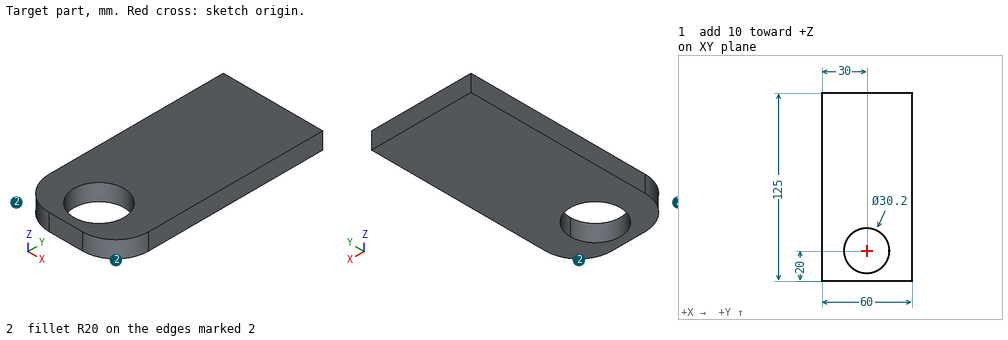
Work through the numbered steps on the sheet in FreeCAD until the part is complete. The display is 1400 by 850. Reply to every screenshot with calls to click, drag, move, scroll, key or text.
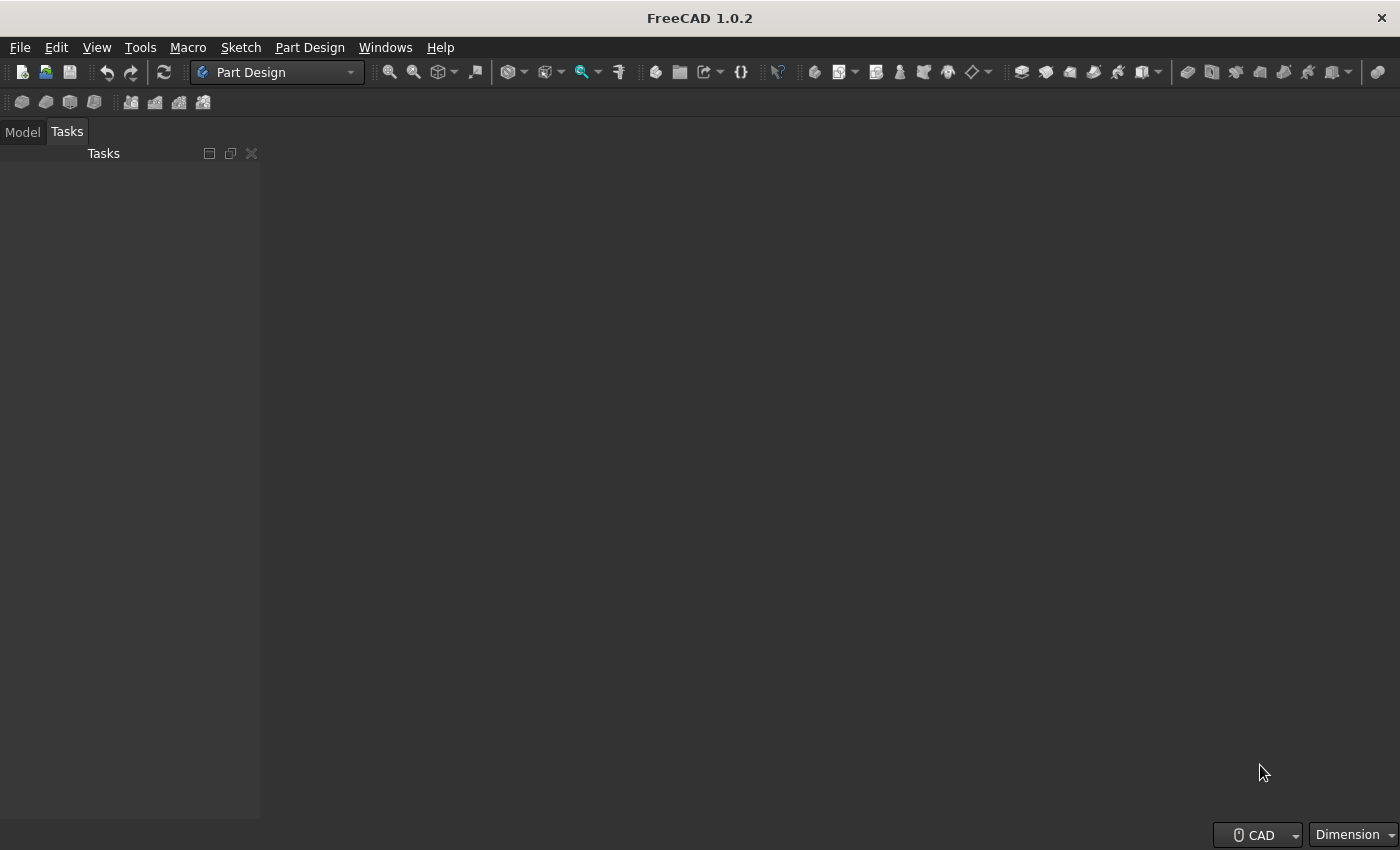
key(ctrl+n)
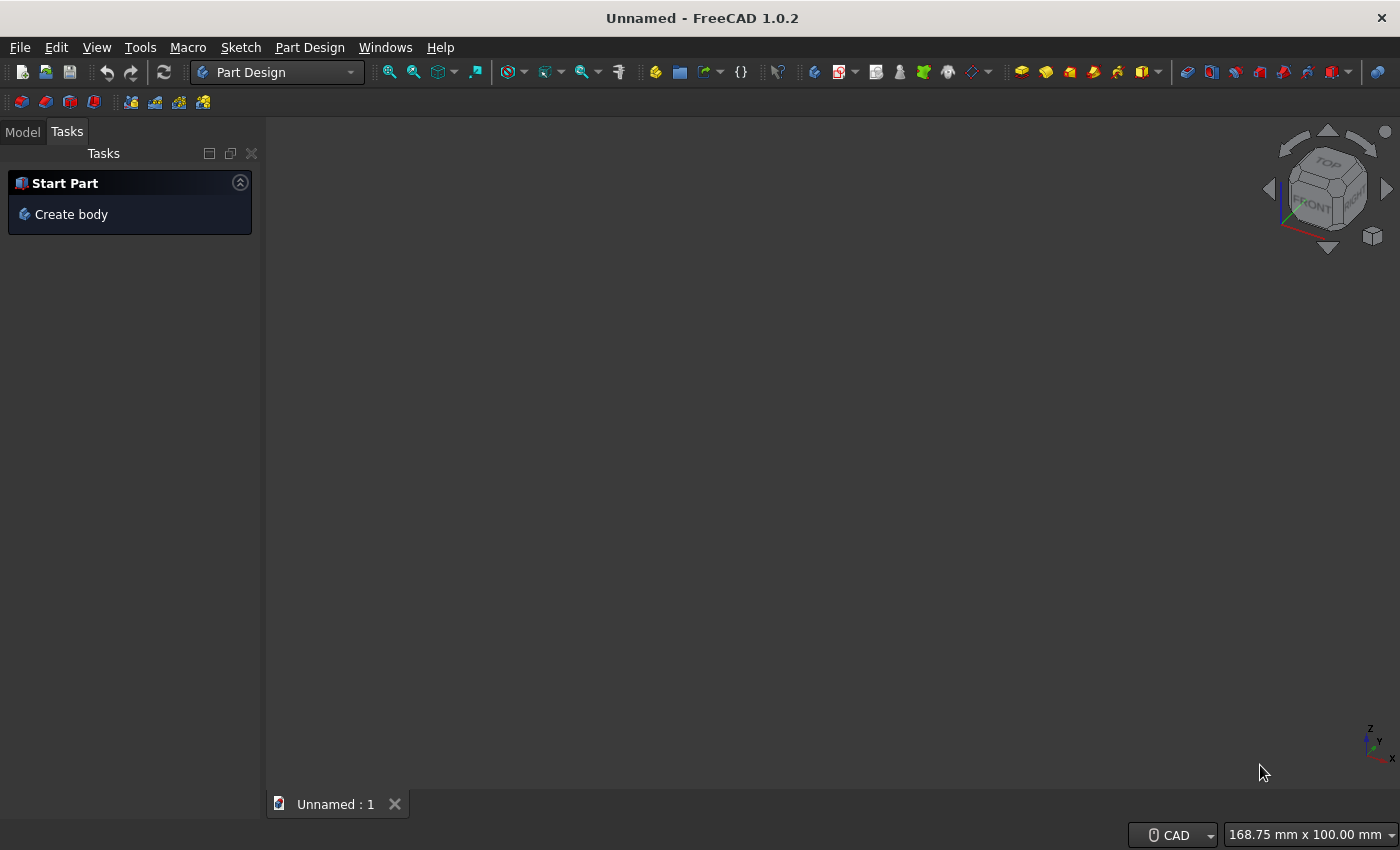
click(840, 72)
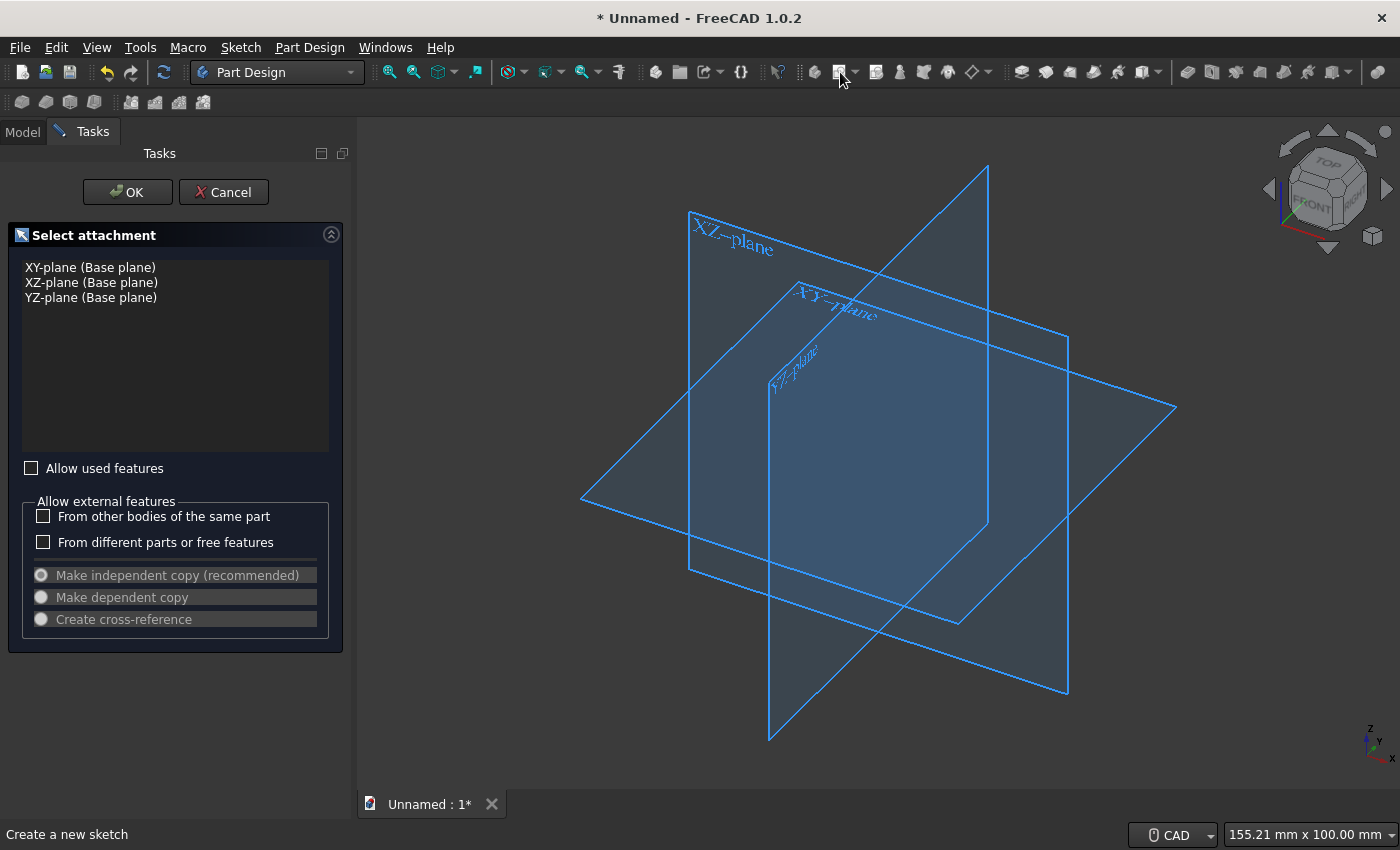
click(82, 268)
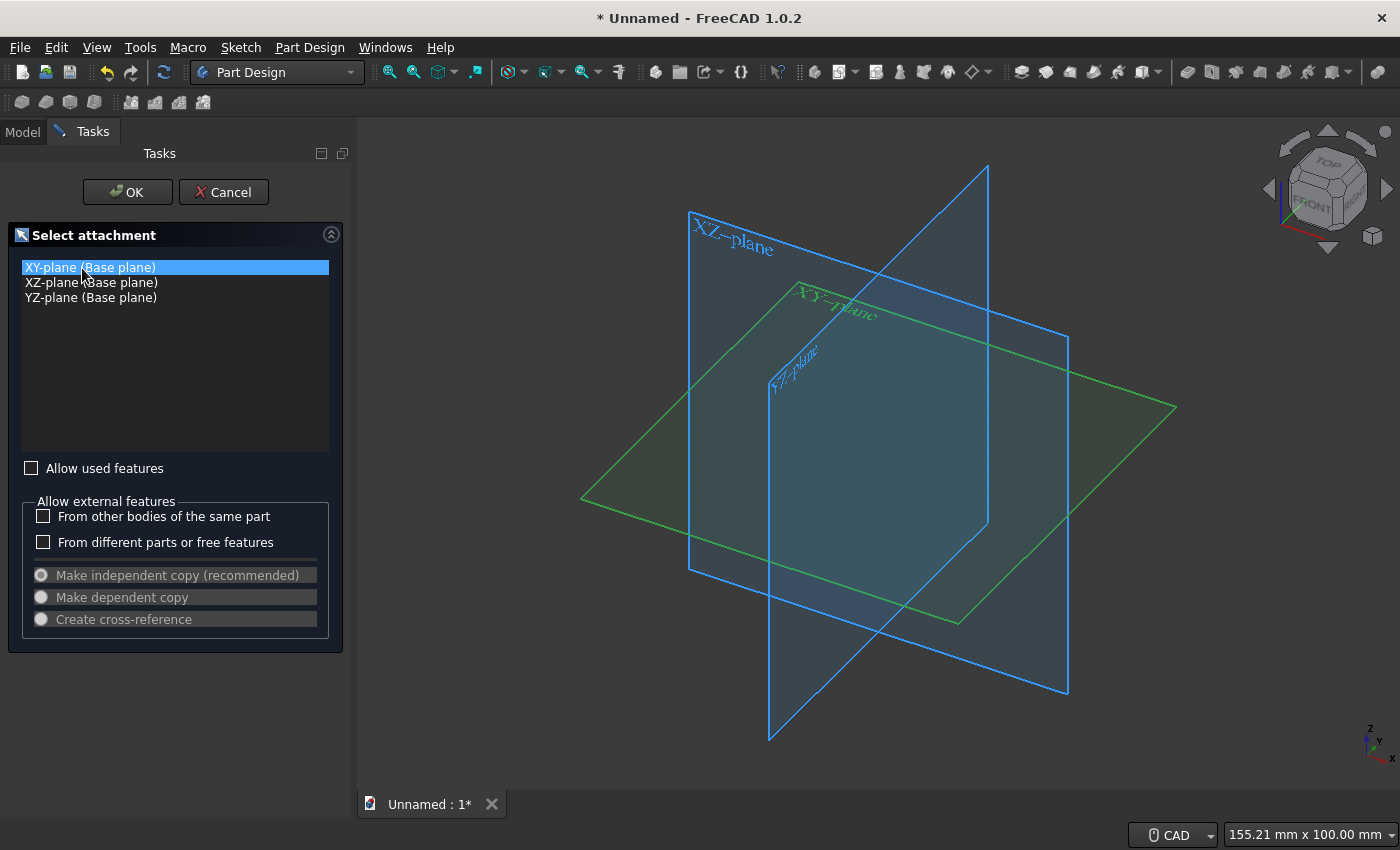
click(128, 192)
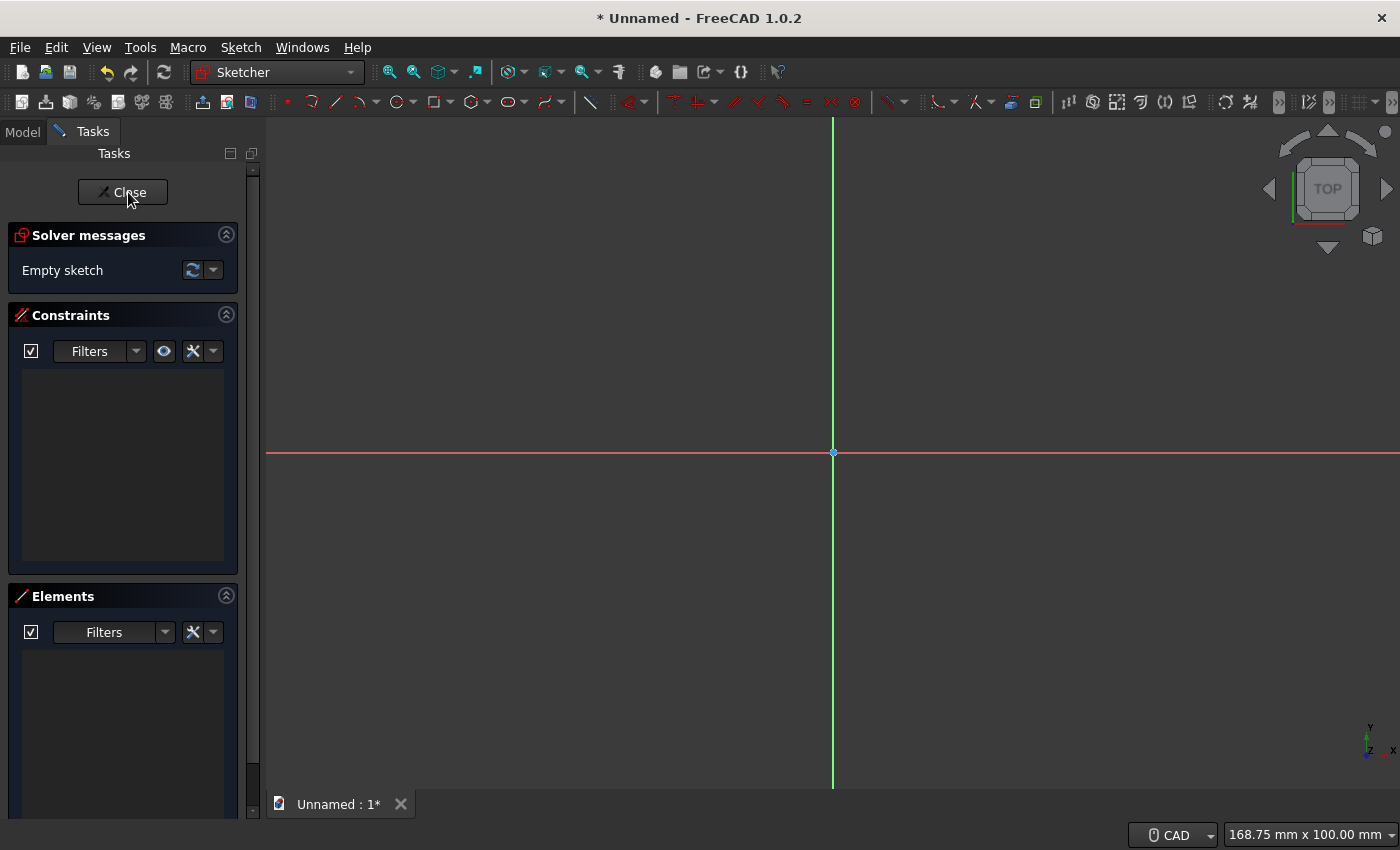
scroll(681, 761, down, 3)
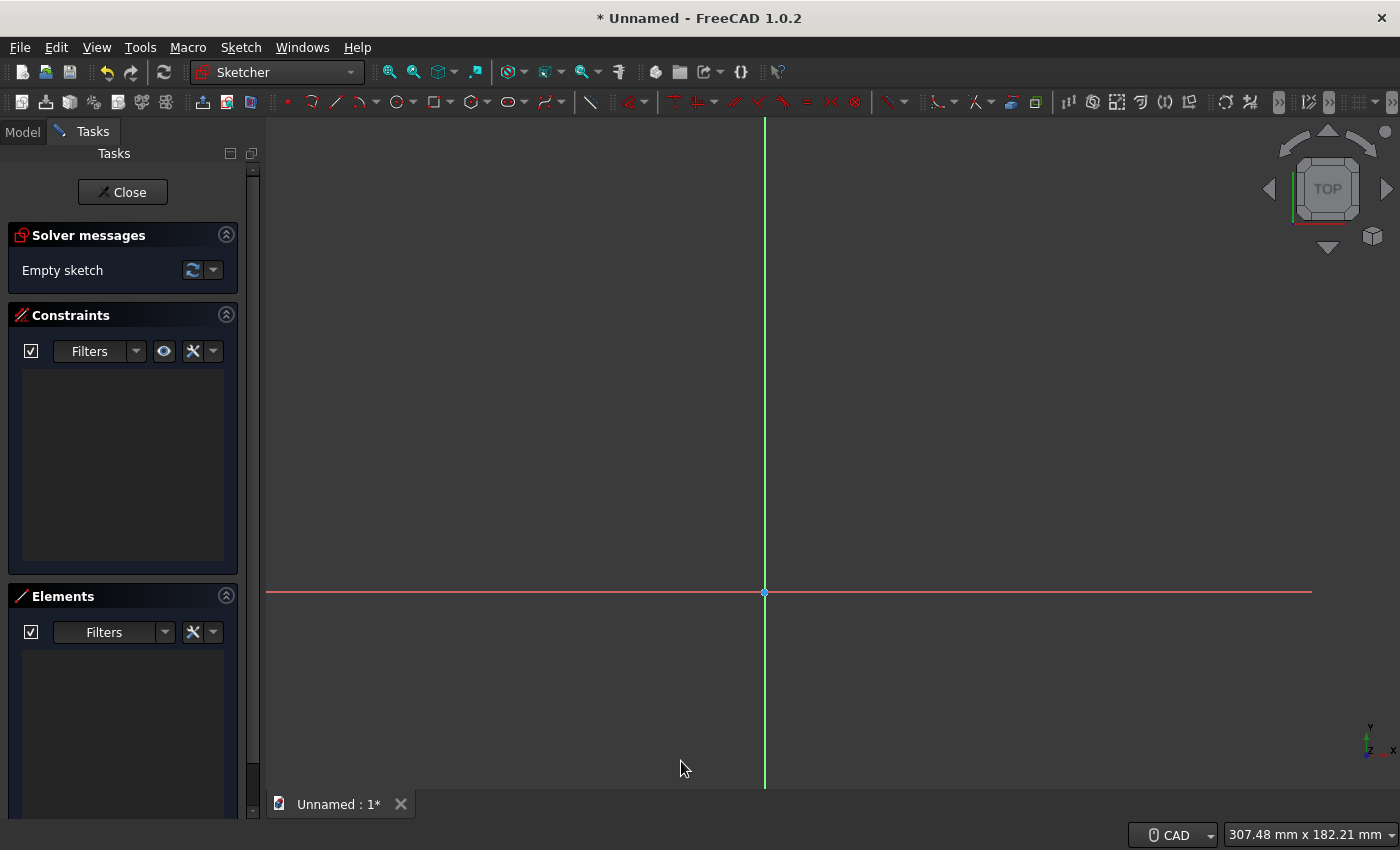
click(434, 102)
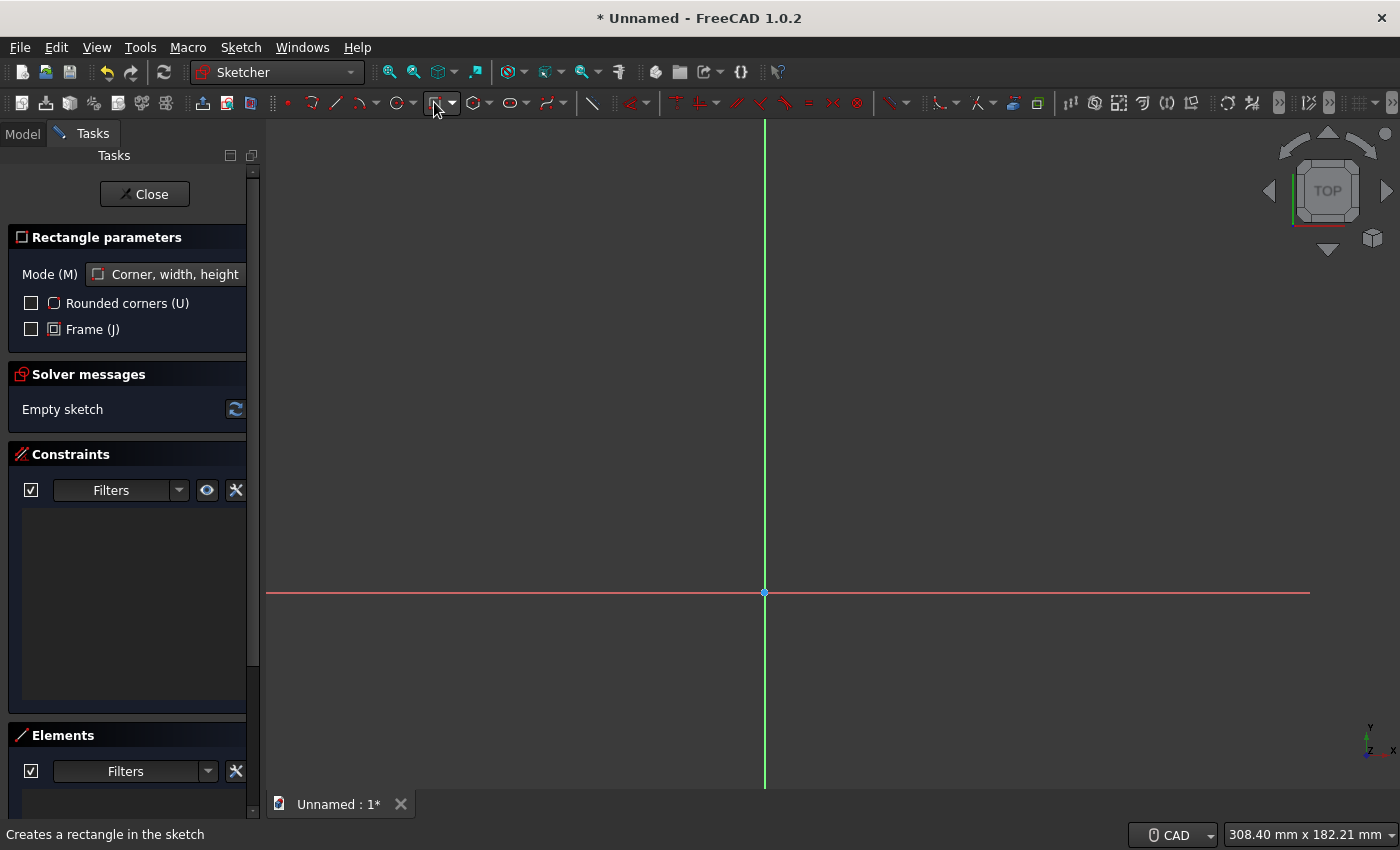
click(654, 207)
click(875, 667)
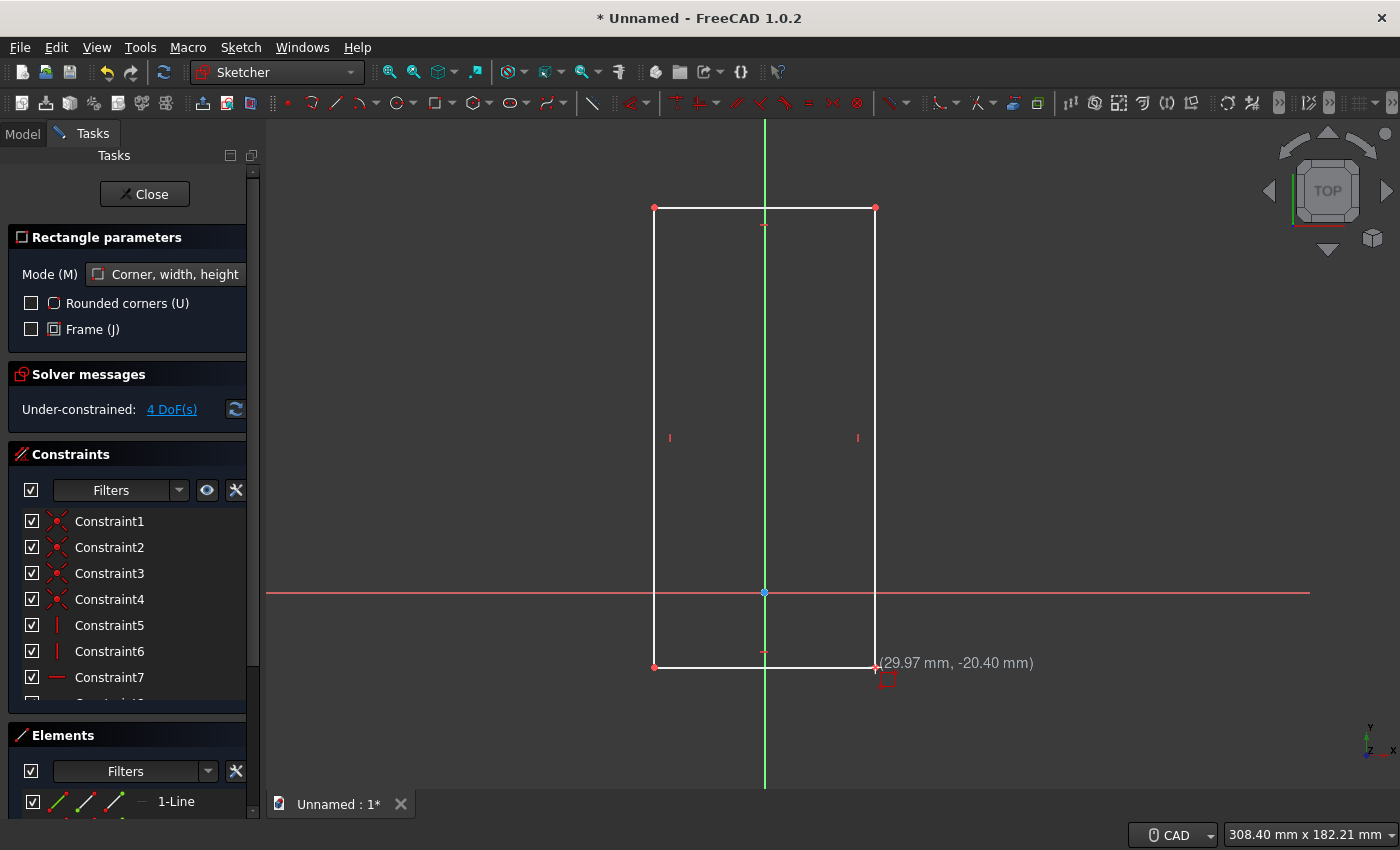
click(398, 104)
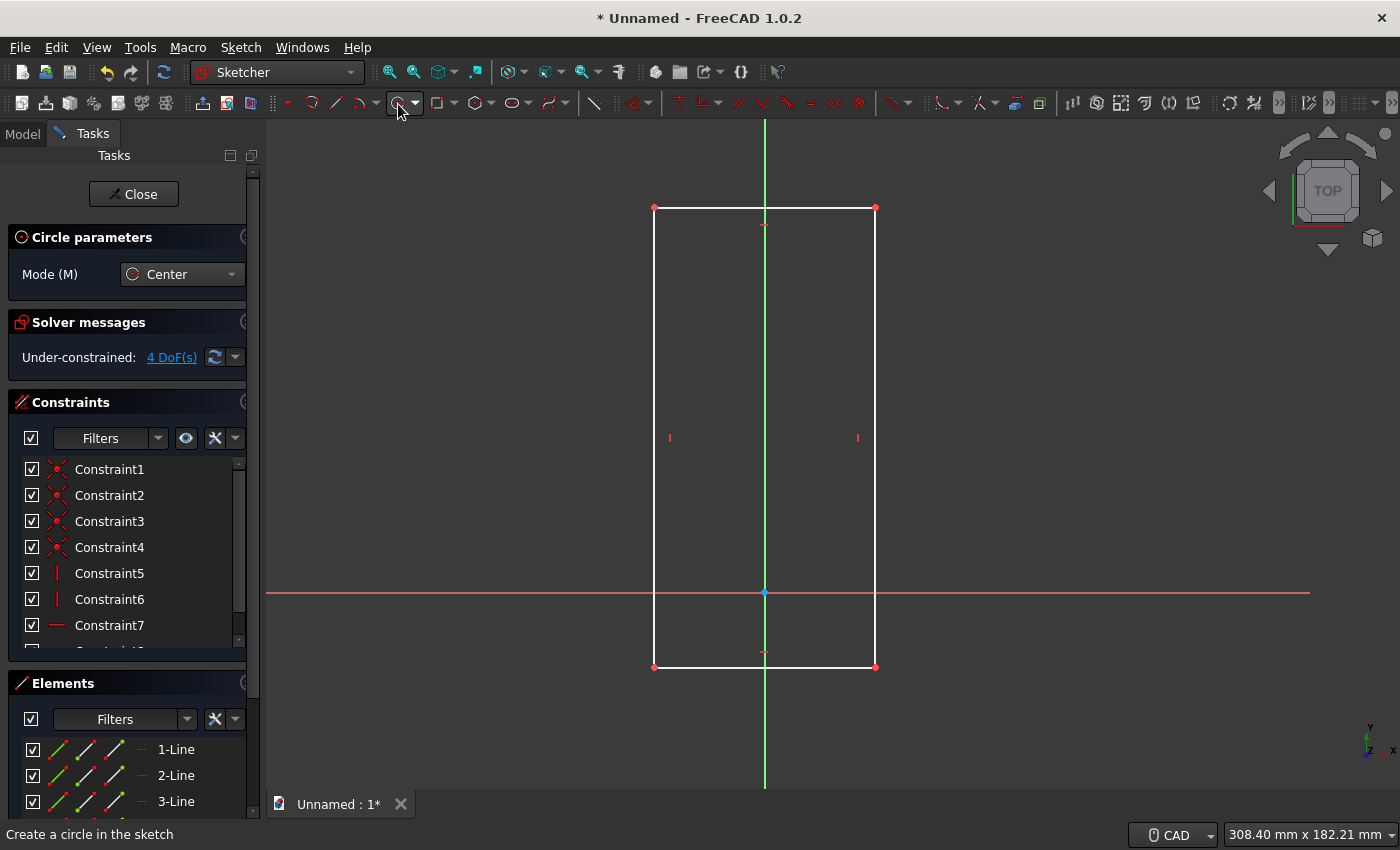
click(765, 593)
click(804, 554)
key(Escape)